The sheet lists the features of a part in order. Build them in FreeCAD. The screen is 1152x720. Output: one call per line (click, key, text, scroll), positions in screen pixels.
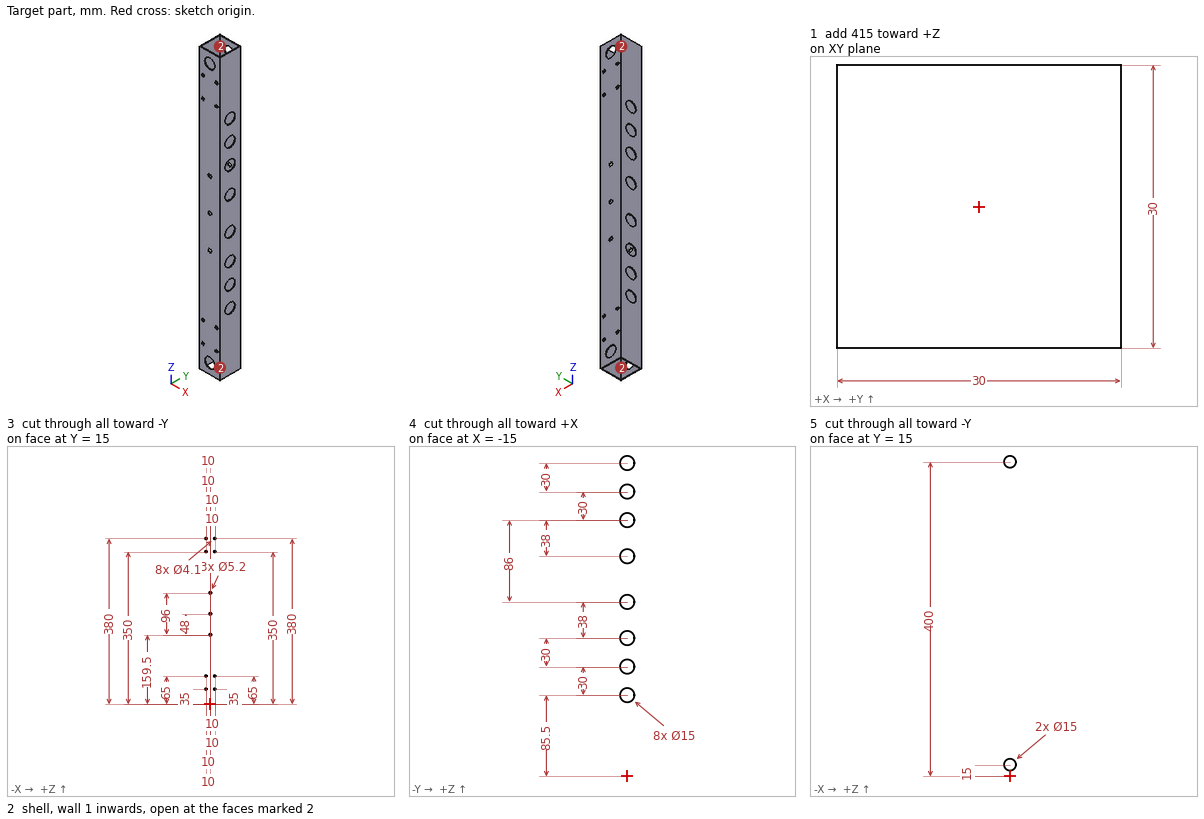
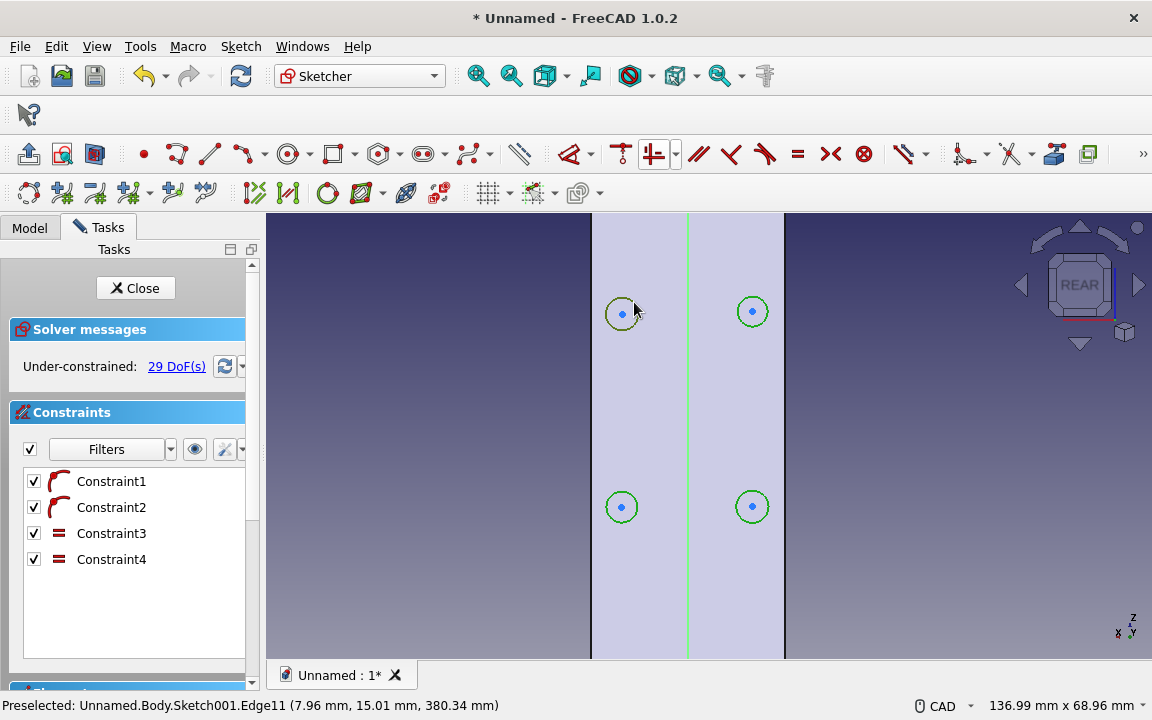
key(e)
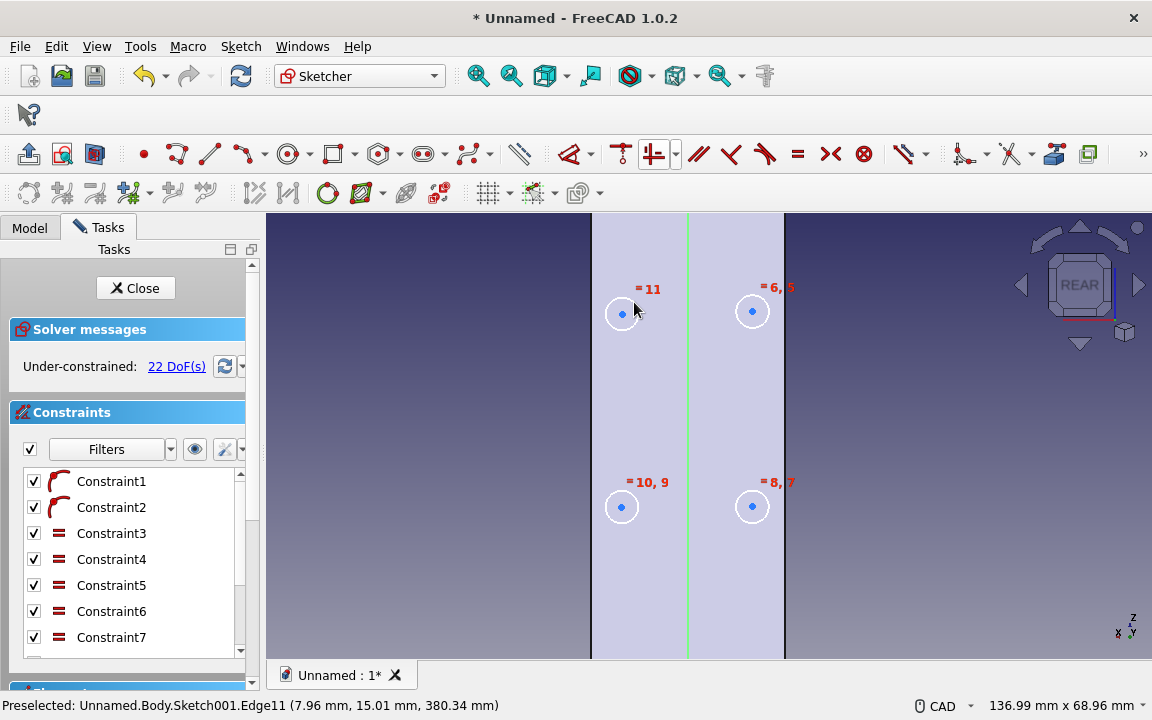
scroll(635, 300, down, 11)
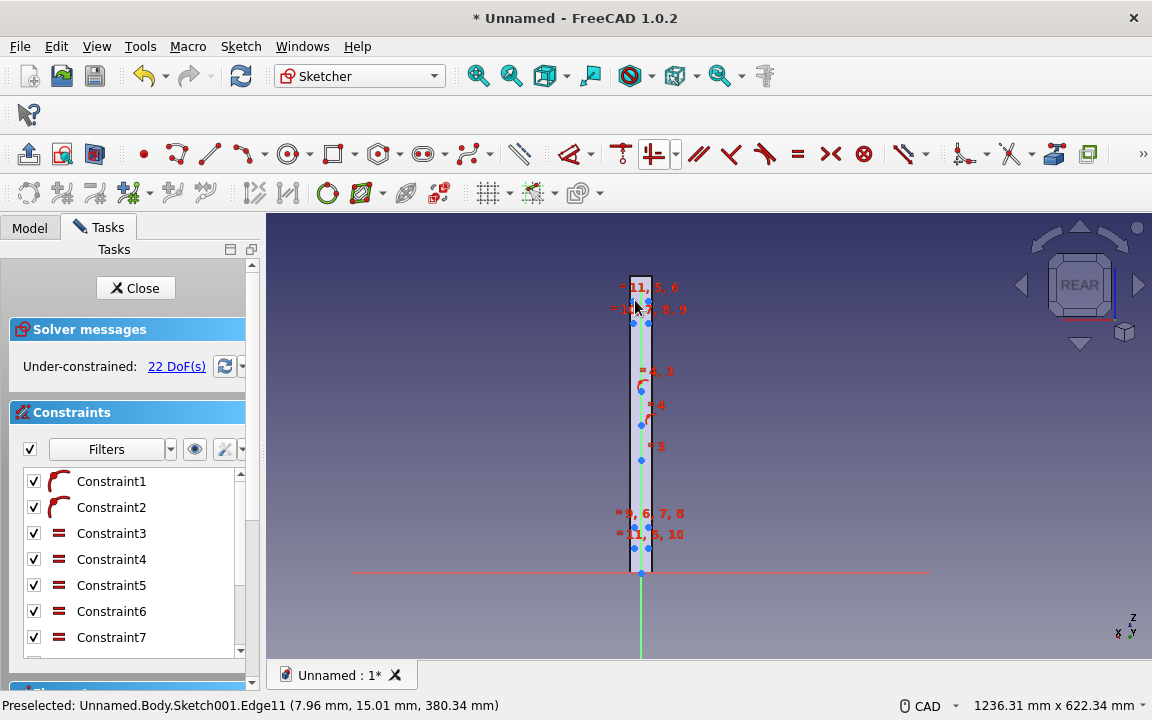
click(642, 460)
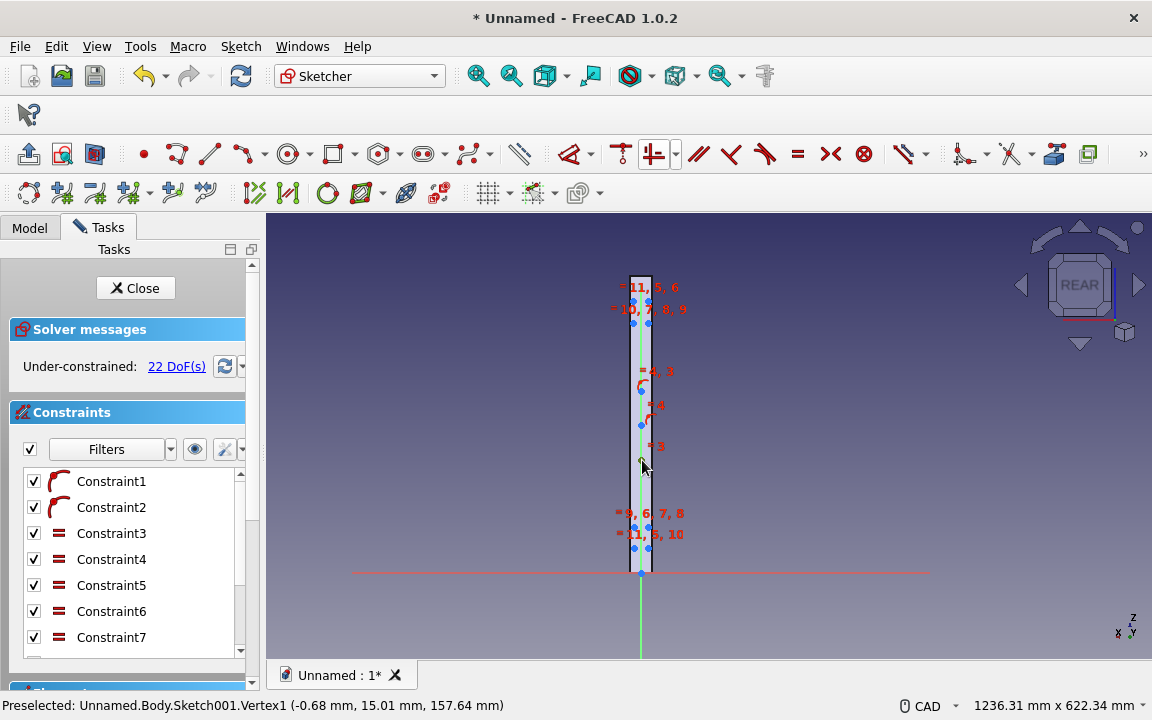
click(641, 603)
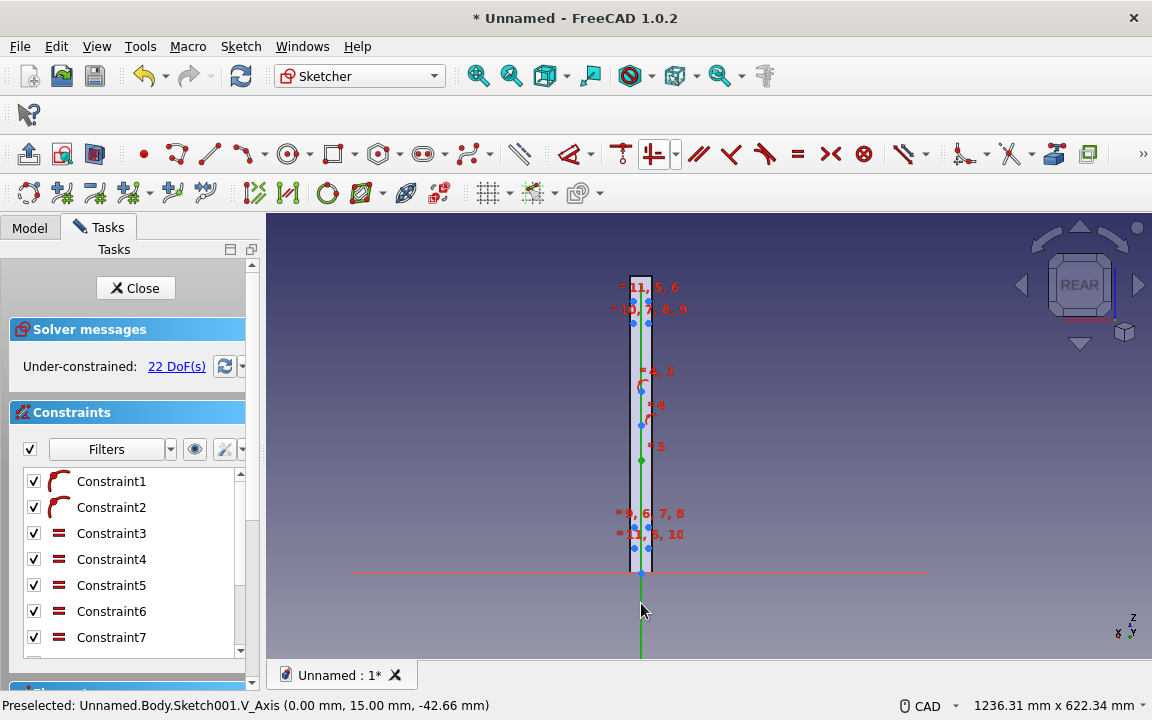
key(c)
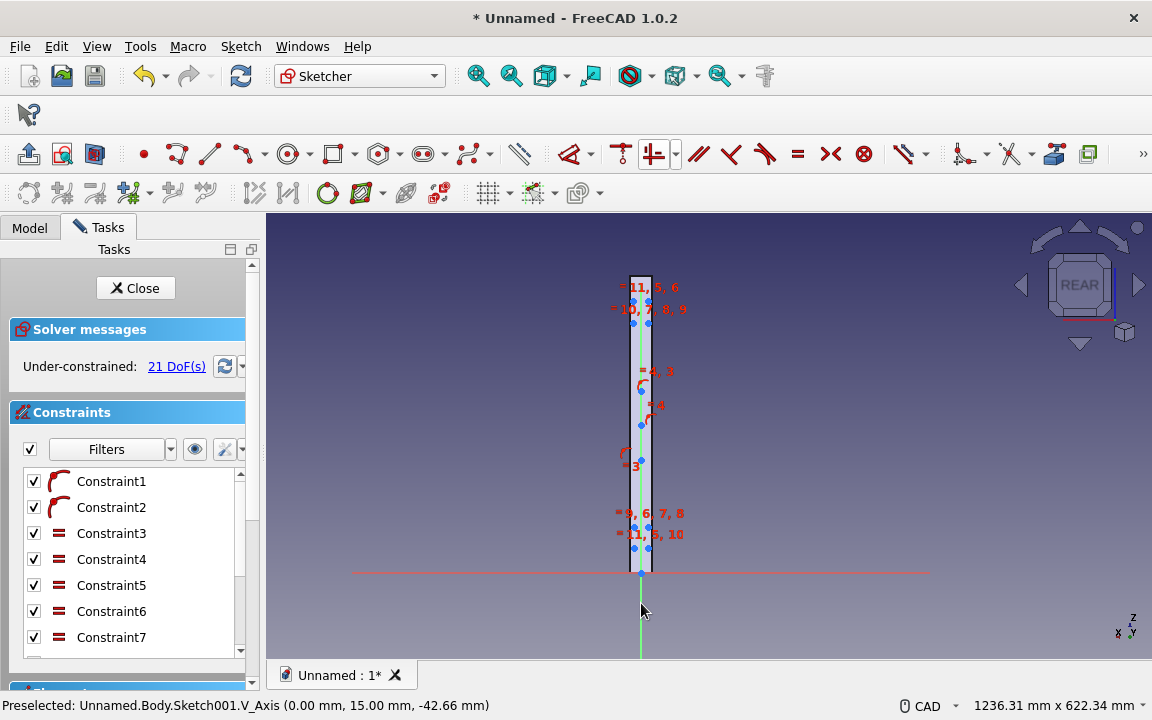
click(568, 154)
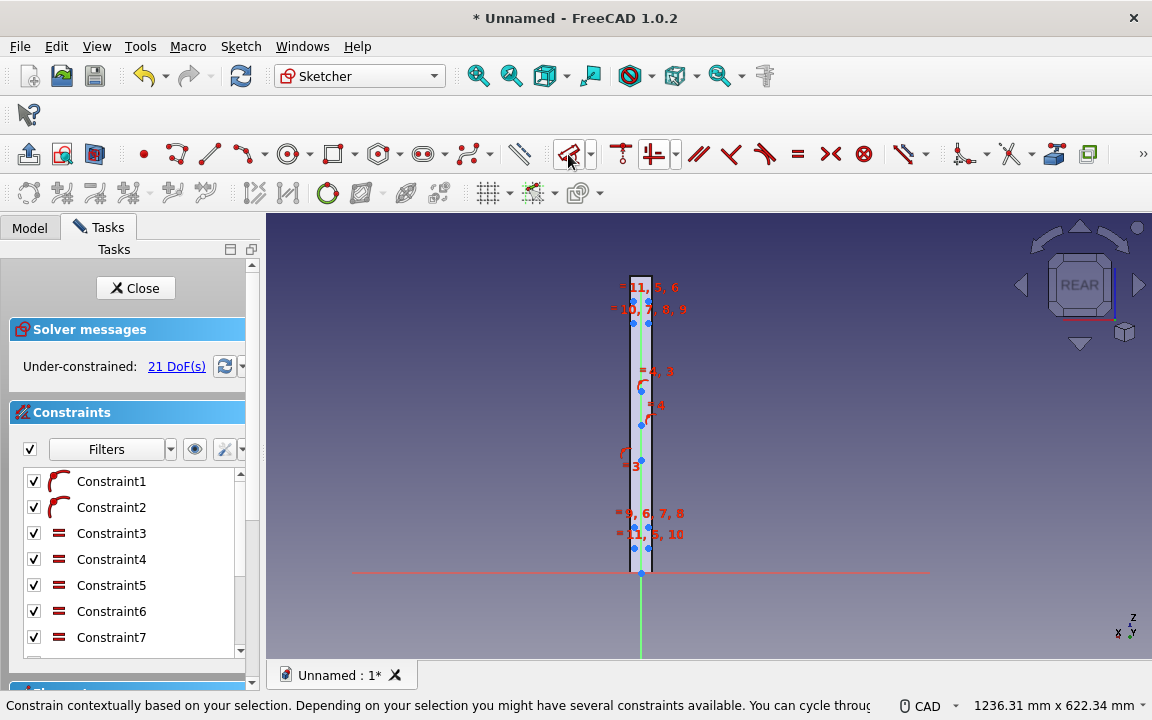
scroll(643, 459, up, 12)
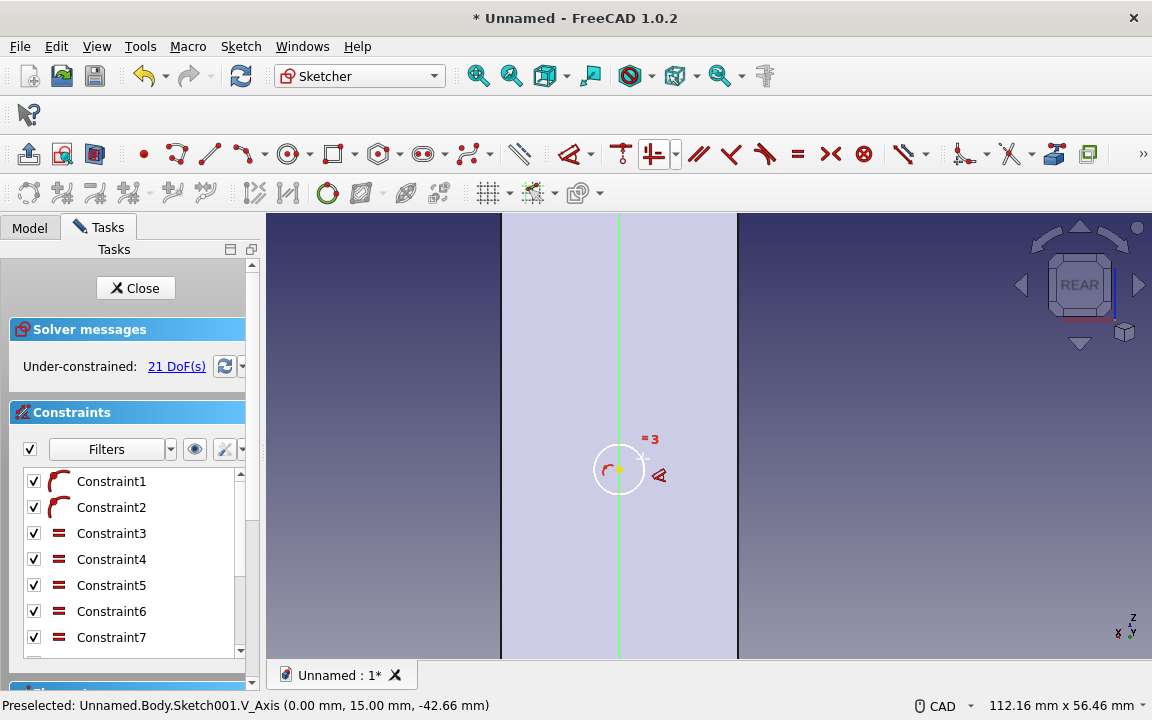
click(637, 452)
click(660, 430)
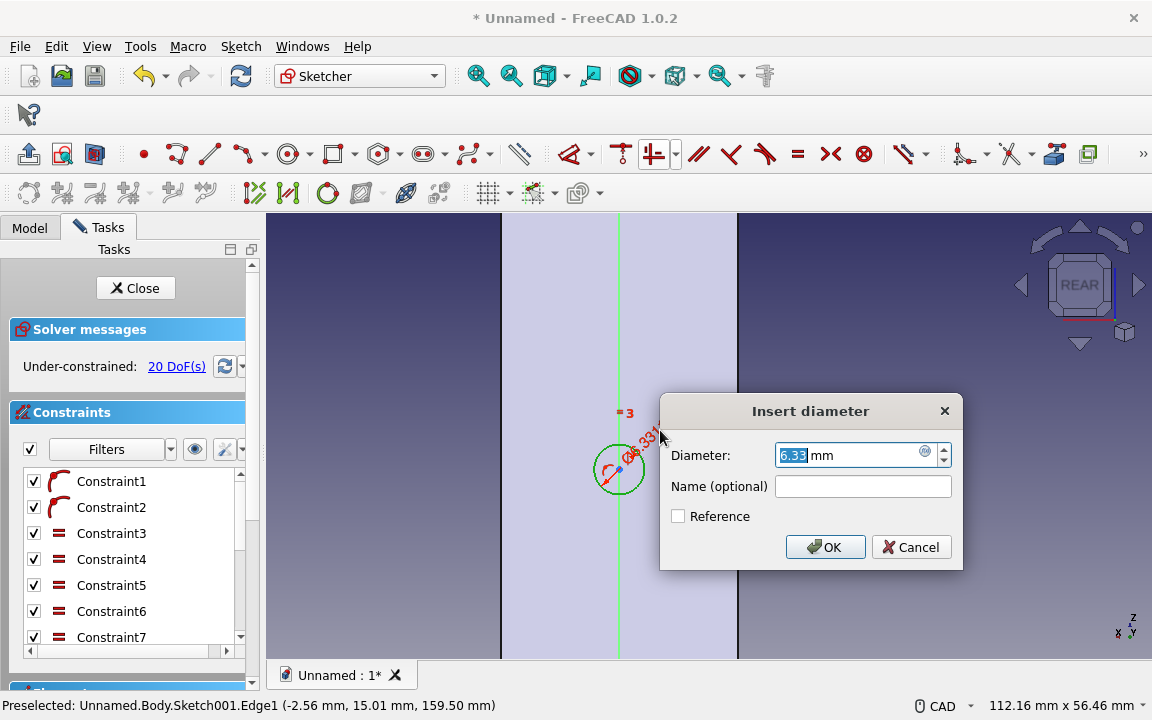
text(5.2)
key(Return)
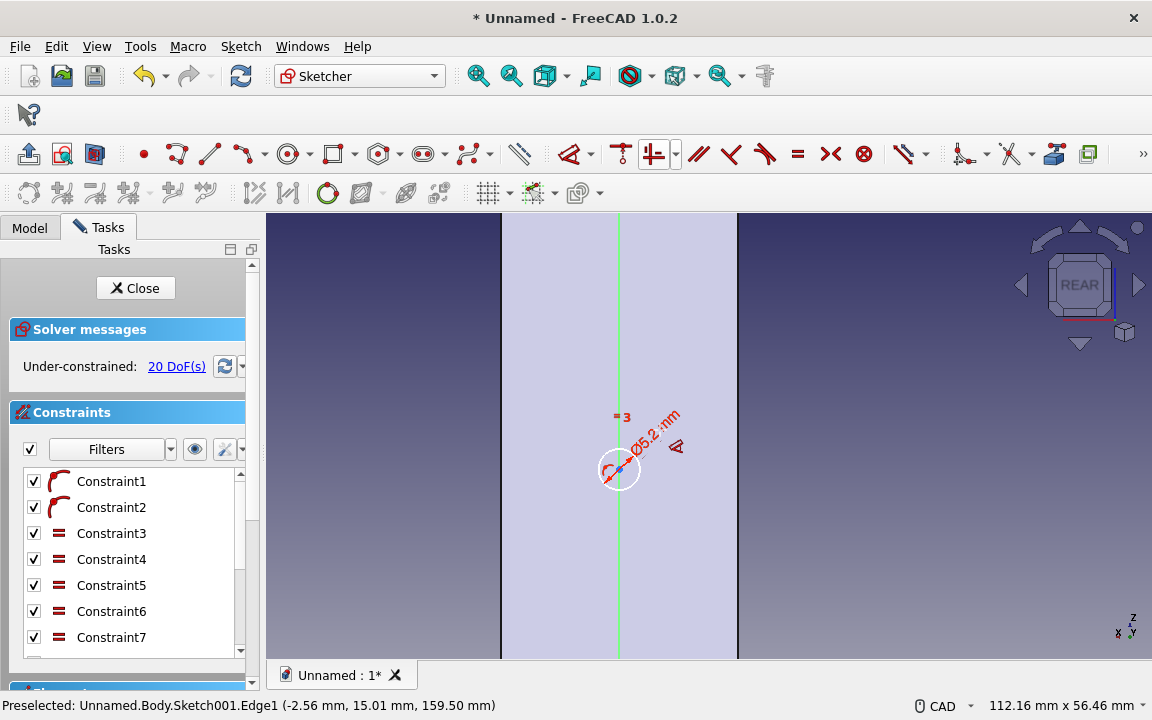
scroll(643, 459, down, 12)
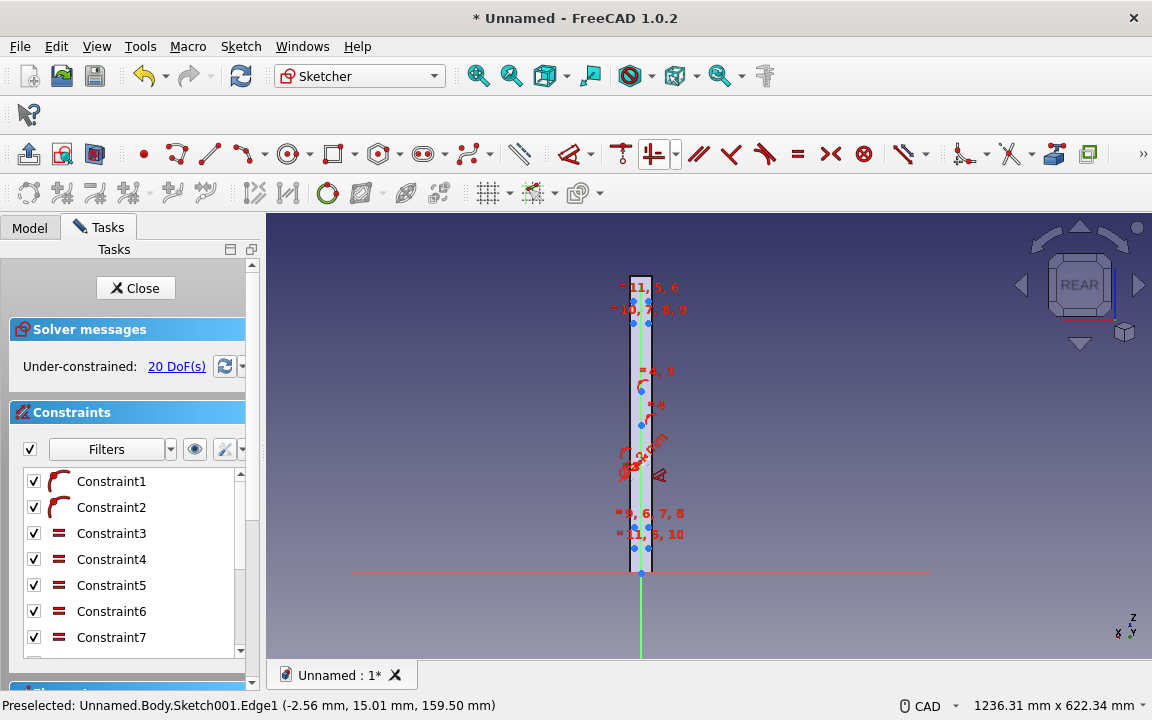
scroll(650, 548, up, 14)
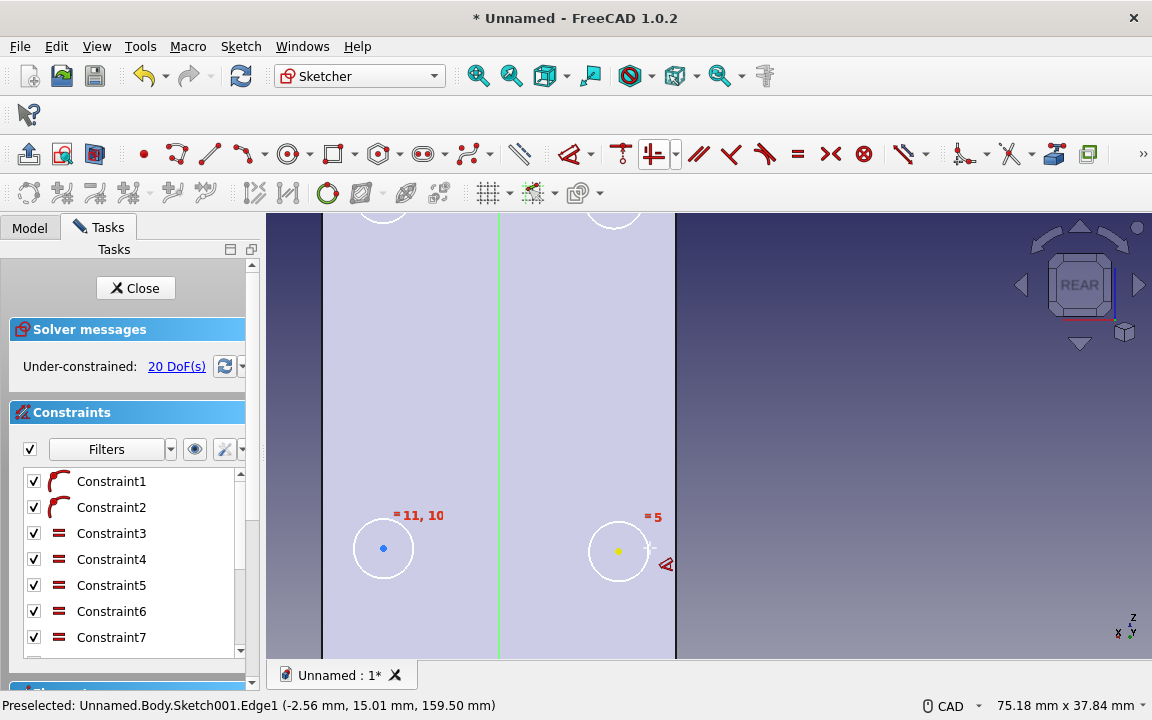
click(640, 531)
click(663, 509)